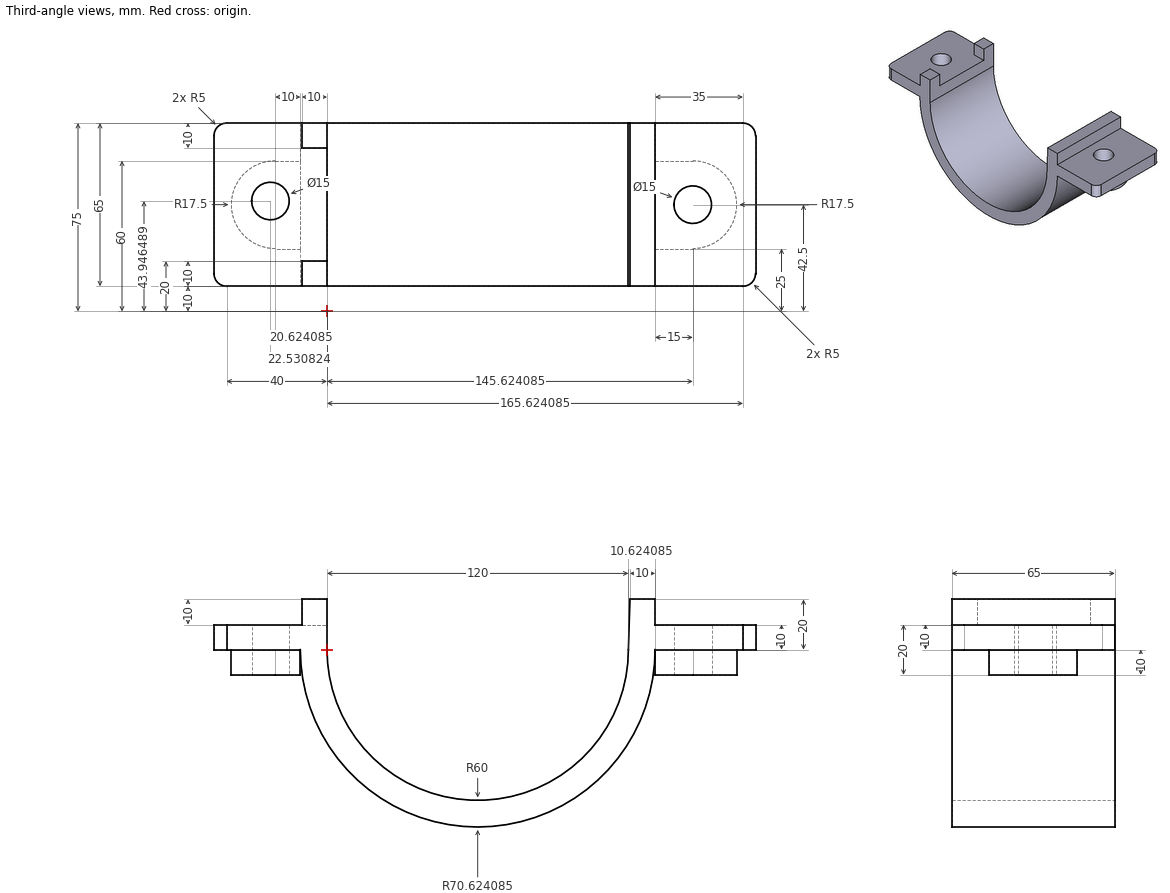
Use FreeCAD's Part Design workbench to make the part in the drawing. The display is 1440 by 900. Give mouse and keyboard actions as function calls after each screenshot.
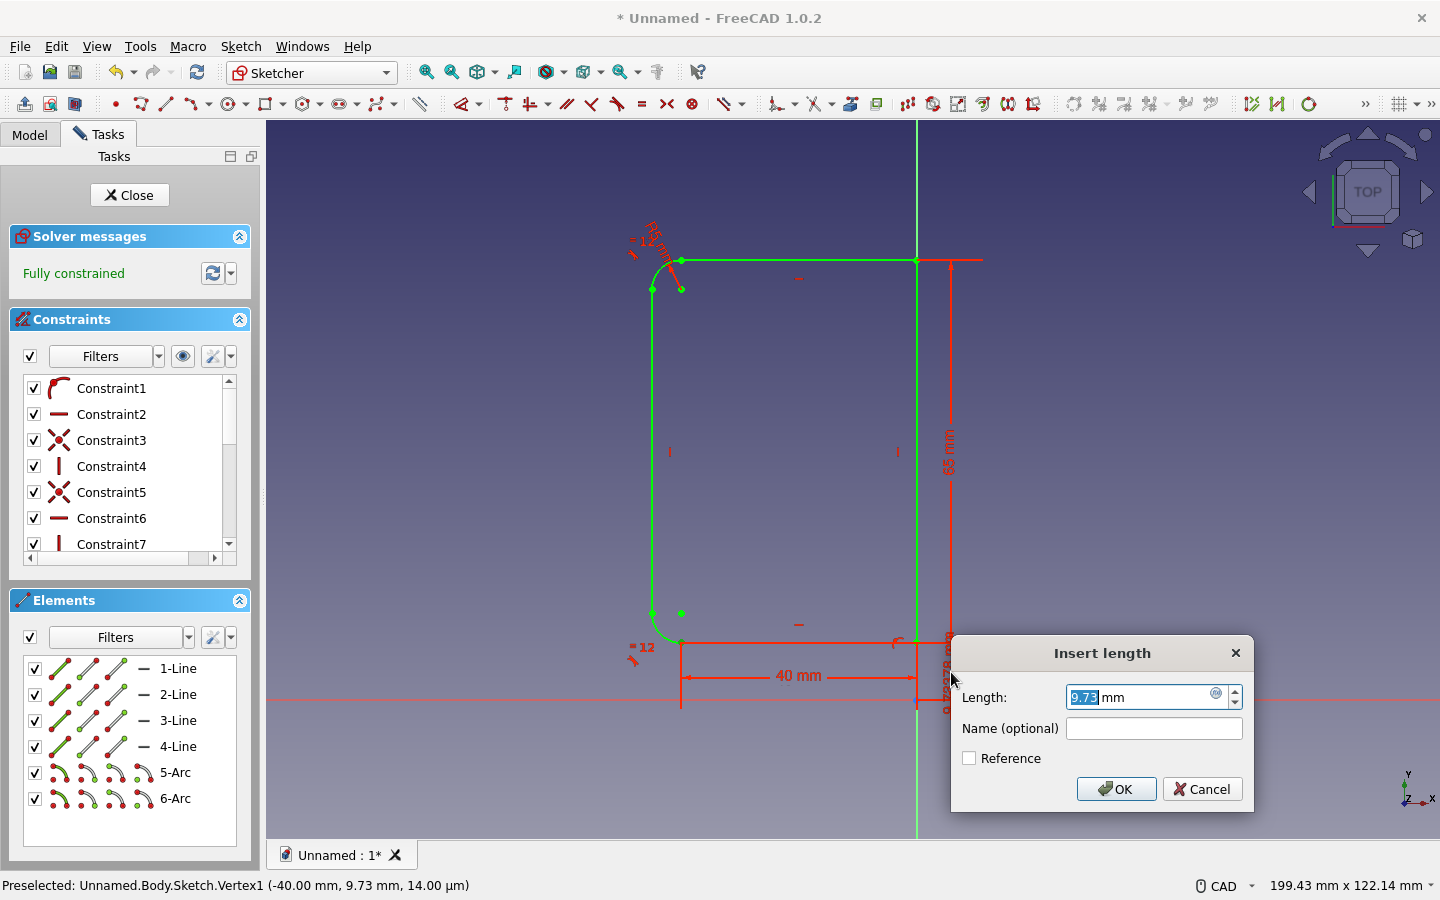
text(10)
key(Return)
key(Escape)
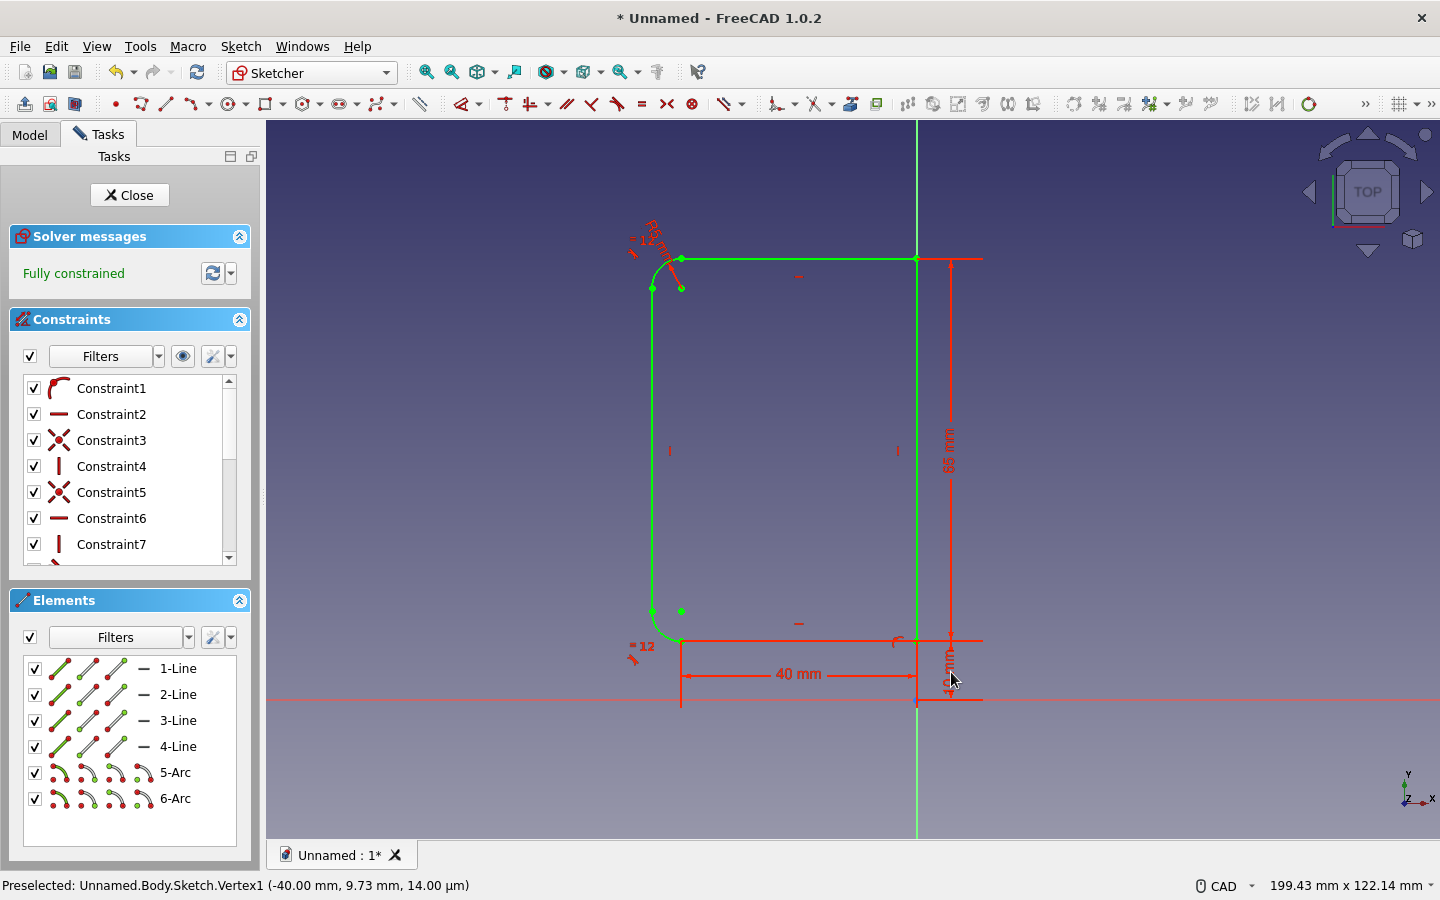
click(130, 195)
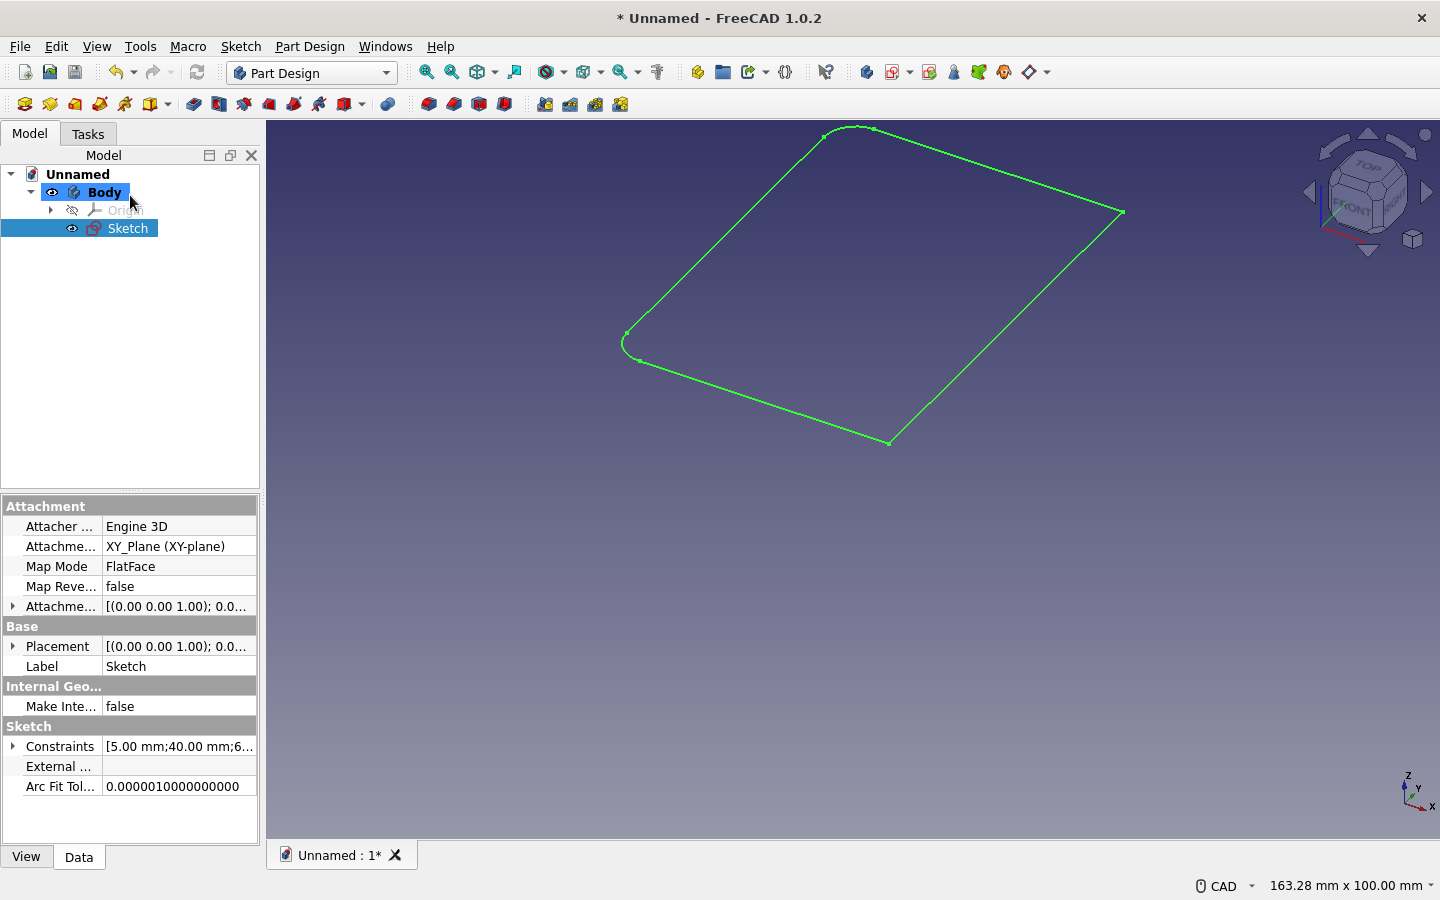
click(25, 104)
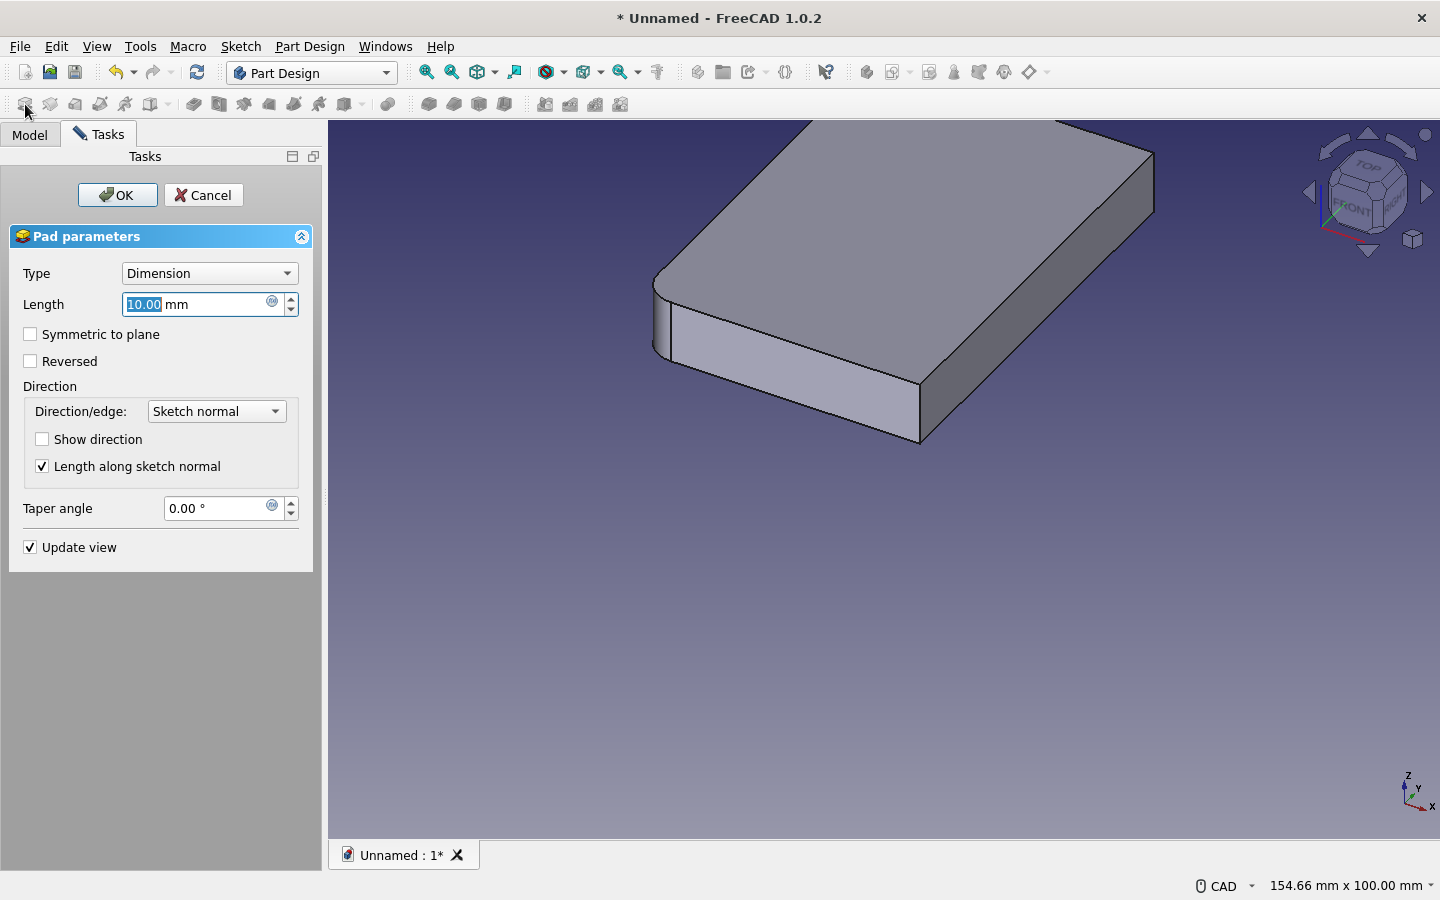
text(10)
key(Tab)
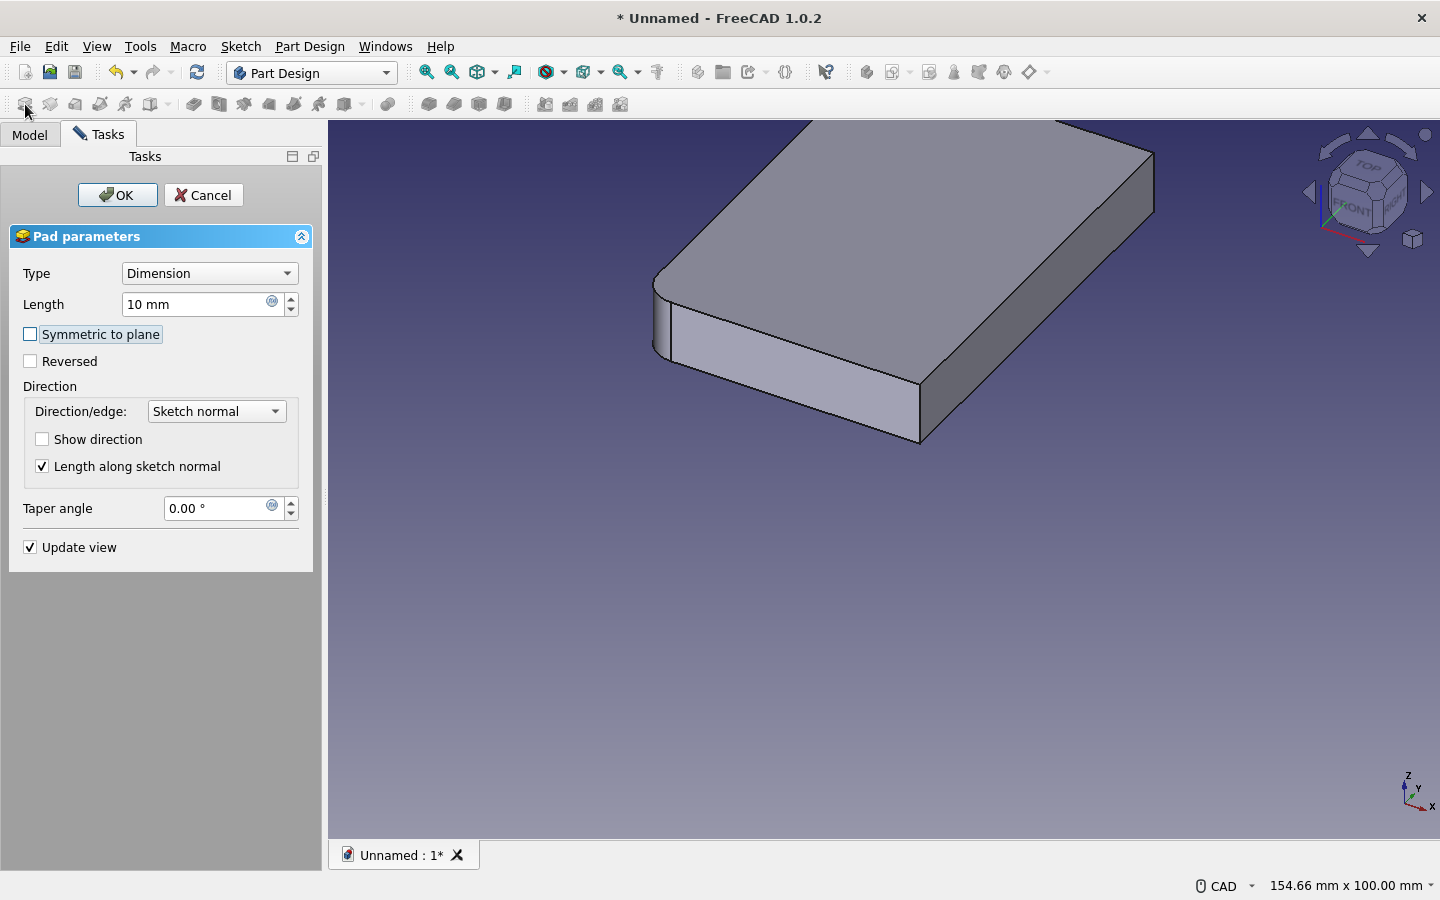
click(118, 195)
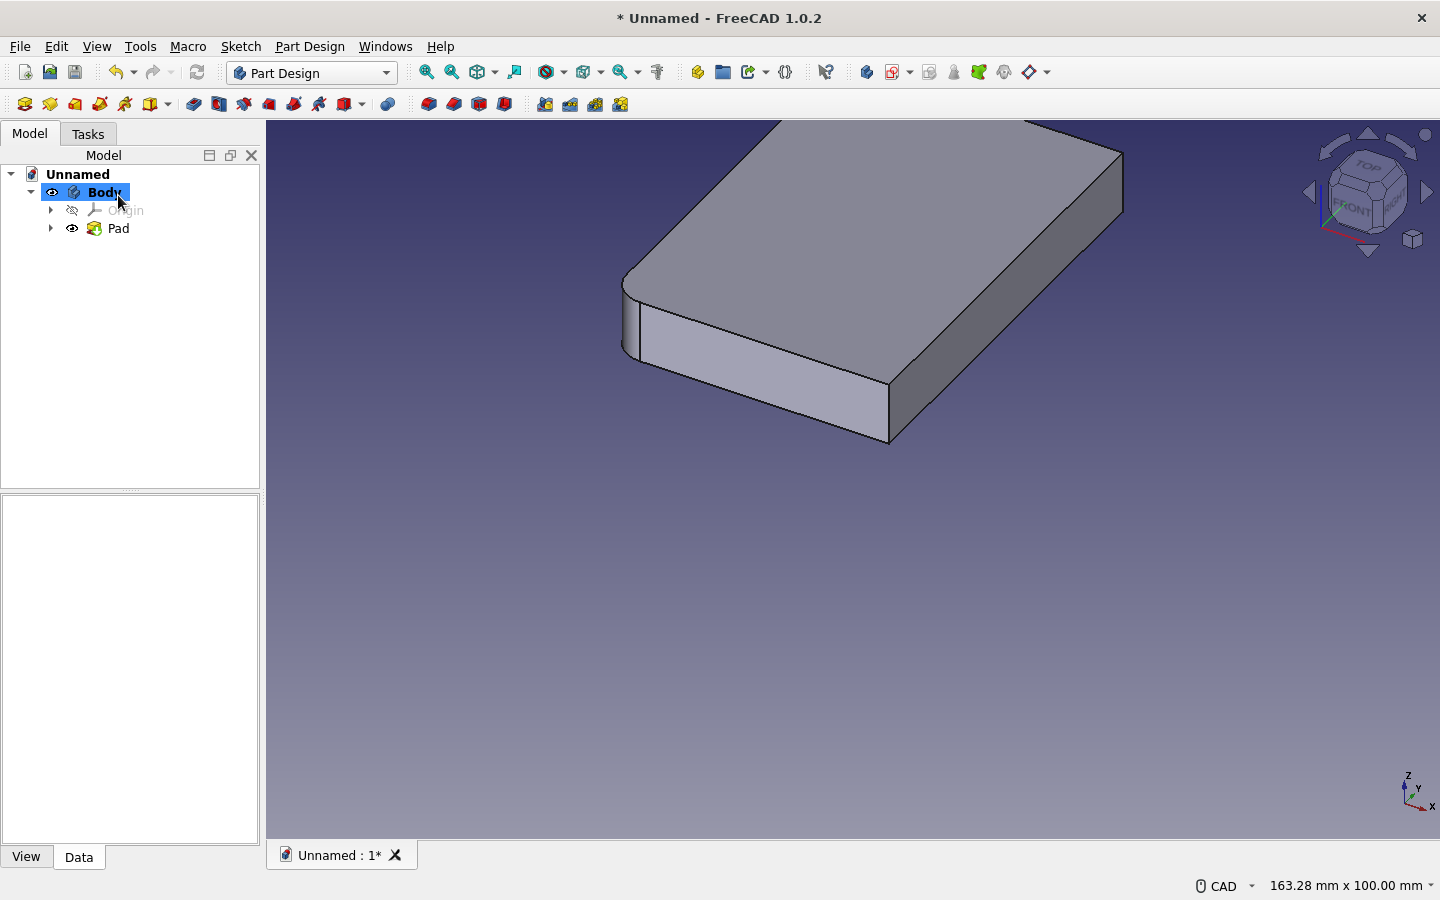
key(v)
key(f)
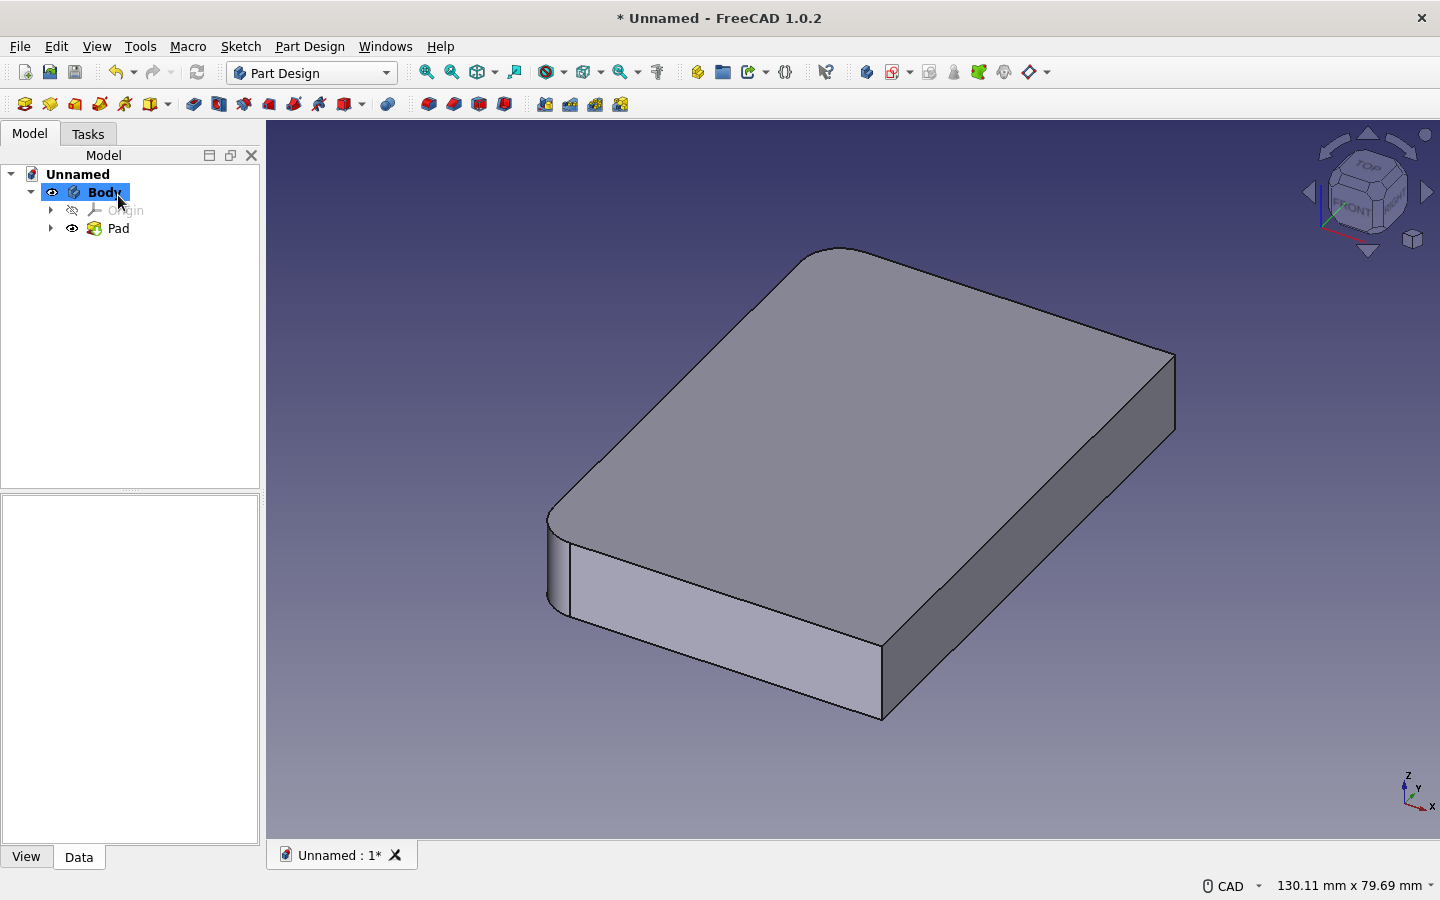
click(895, 400)